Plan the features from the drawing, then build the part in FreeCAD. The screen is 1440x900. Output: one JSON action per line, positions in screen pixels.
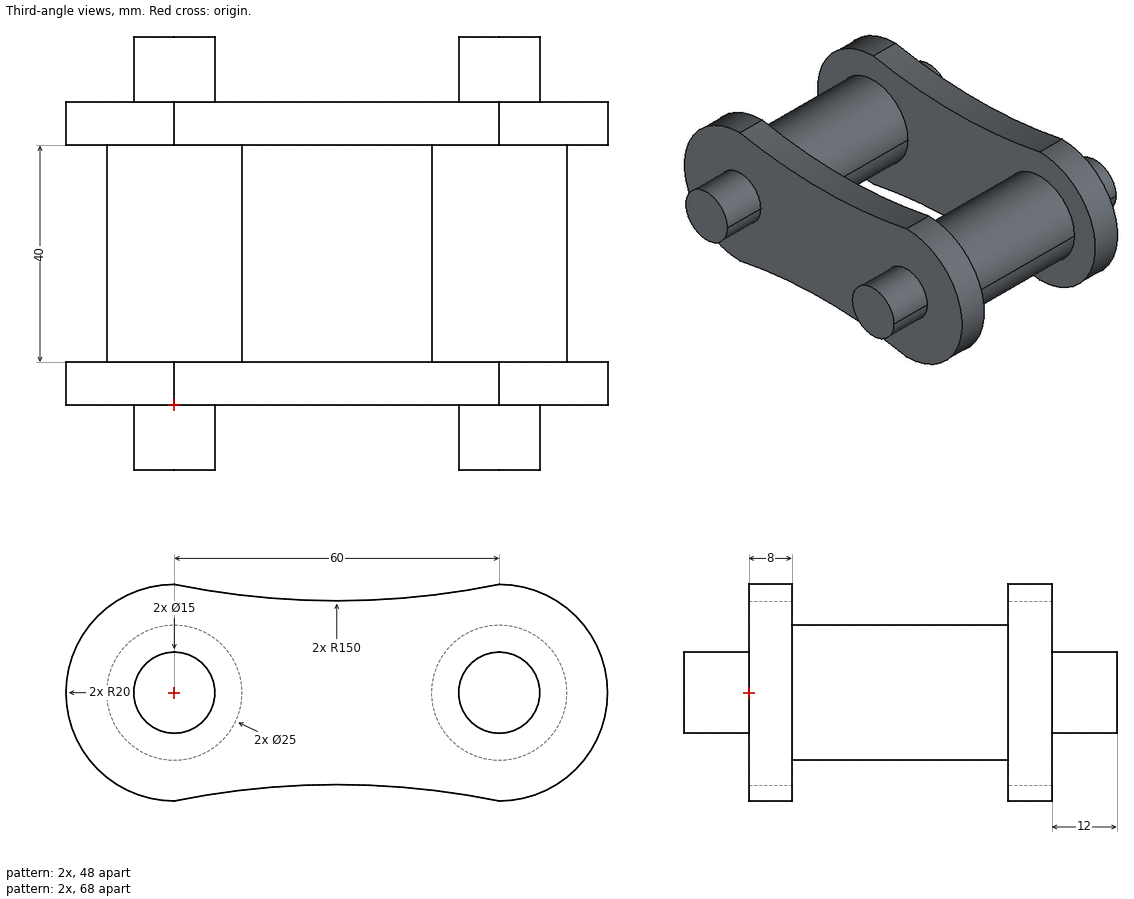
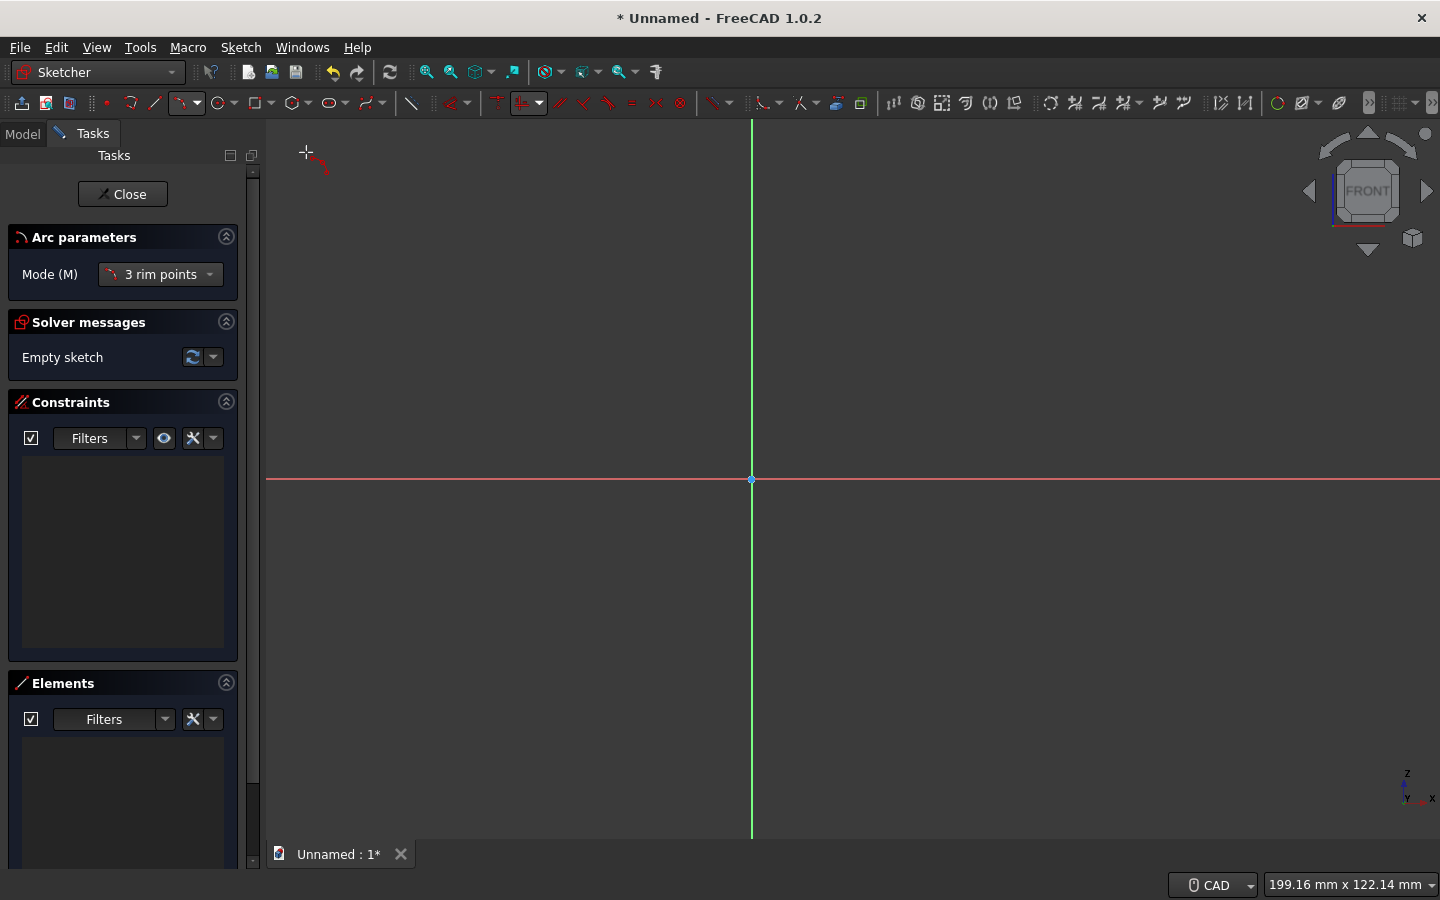
{"action": "left_click", "coordinate": [752, 597]}
{"action": "left_click", "coordinate": [752, 361]}
{"action": "left_click", "coordinate": [640, 443]}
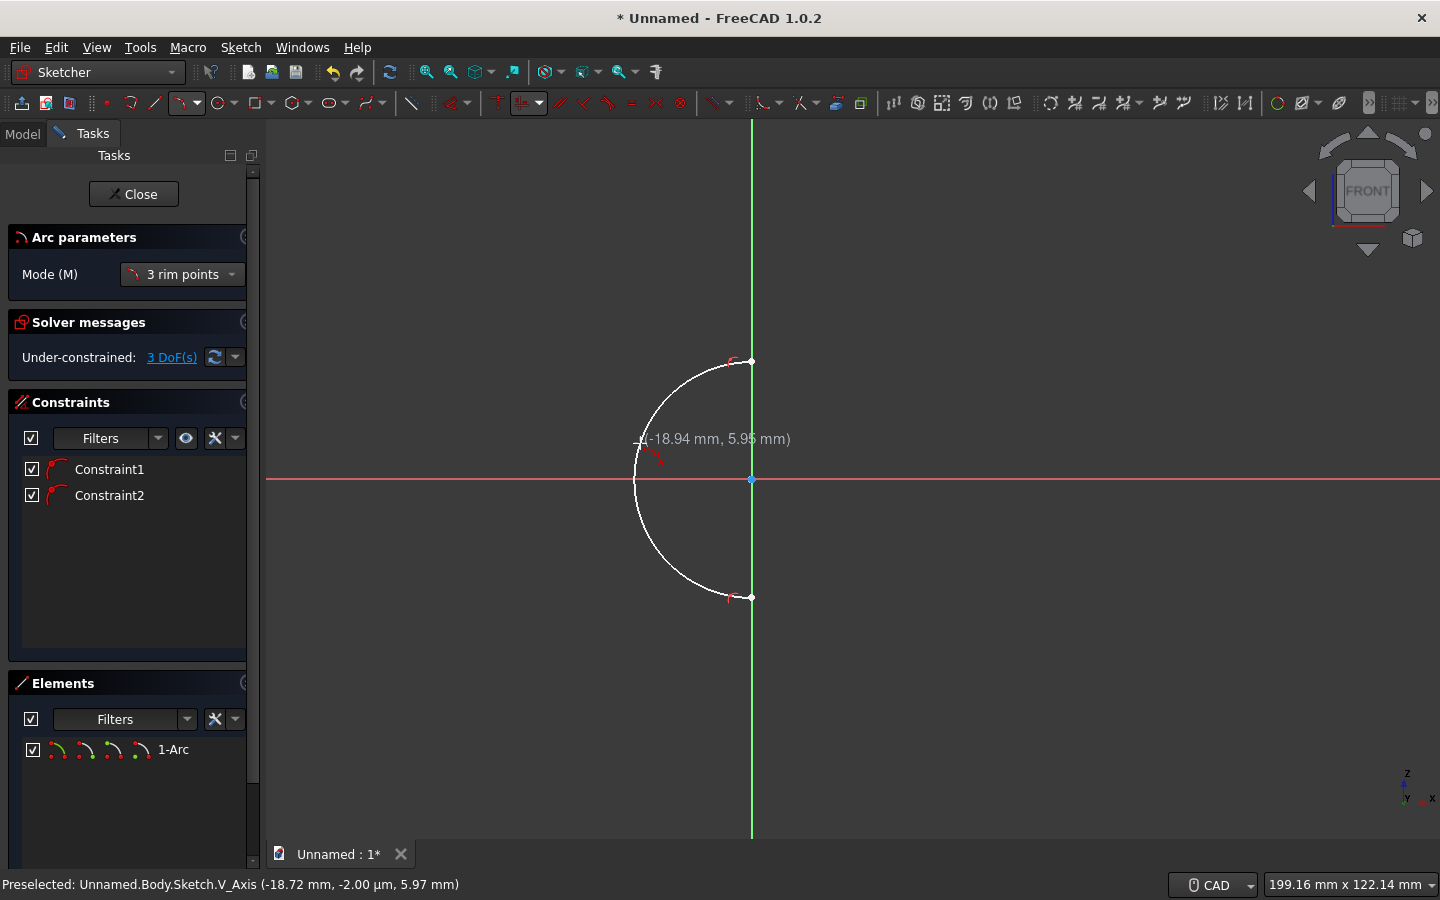
{"action": "left_click", "coordinate": [752, 362]}
{"action": "left_click", "coordinate": [1105, 361]}
{"action": "left_click", "coordinate": [929, 379]}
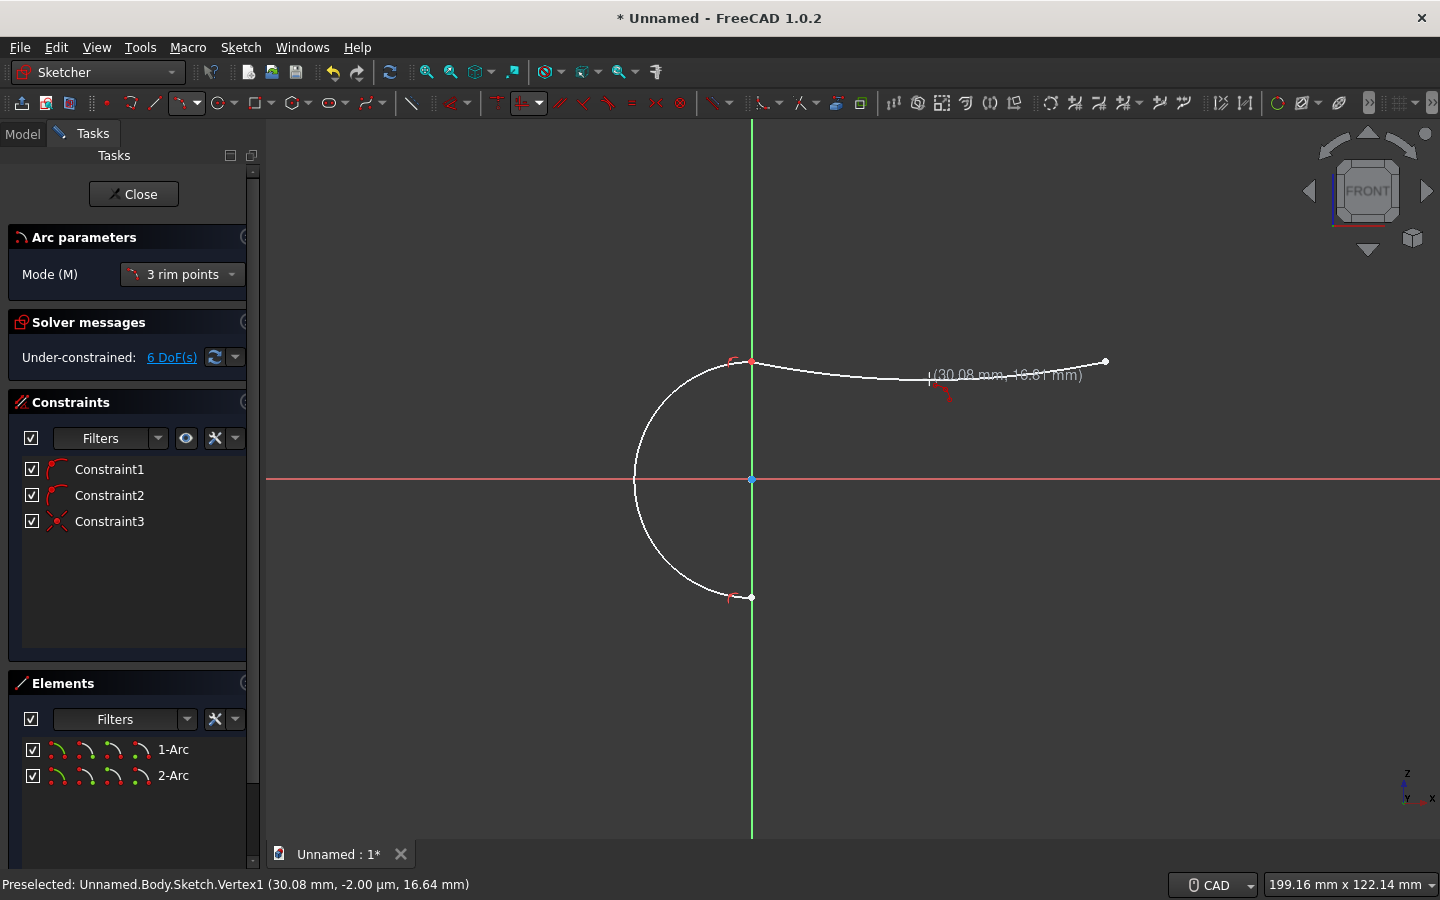
{"action": "left_click", "coordinate": [1105, 362]}
{"action": "left_click", "coordinate": [1105, 597]}
{"action": "left_click", "coordinate": [1217, 516]}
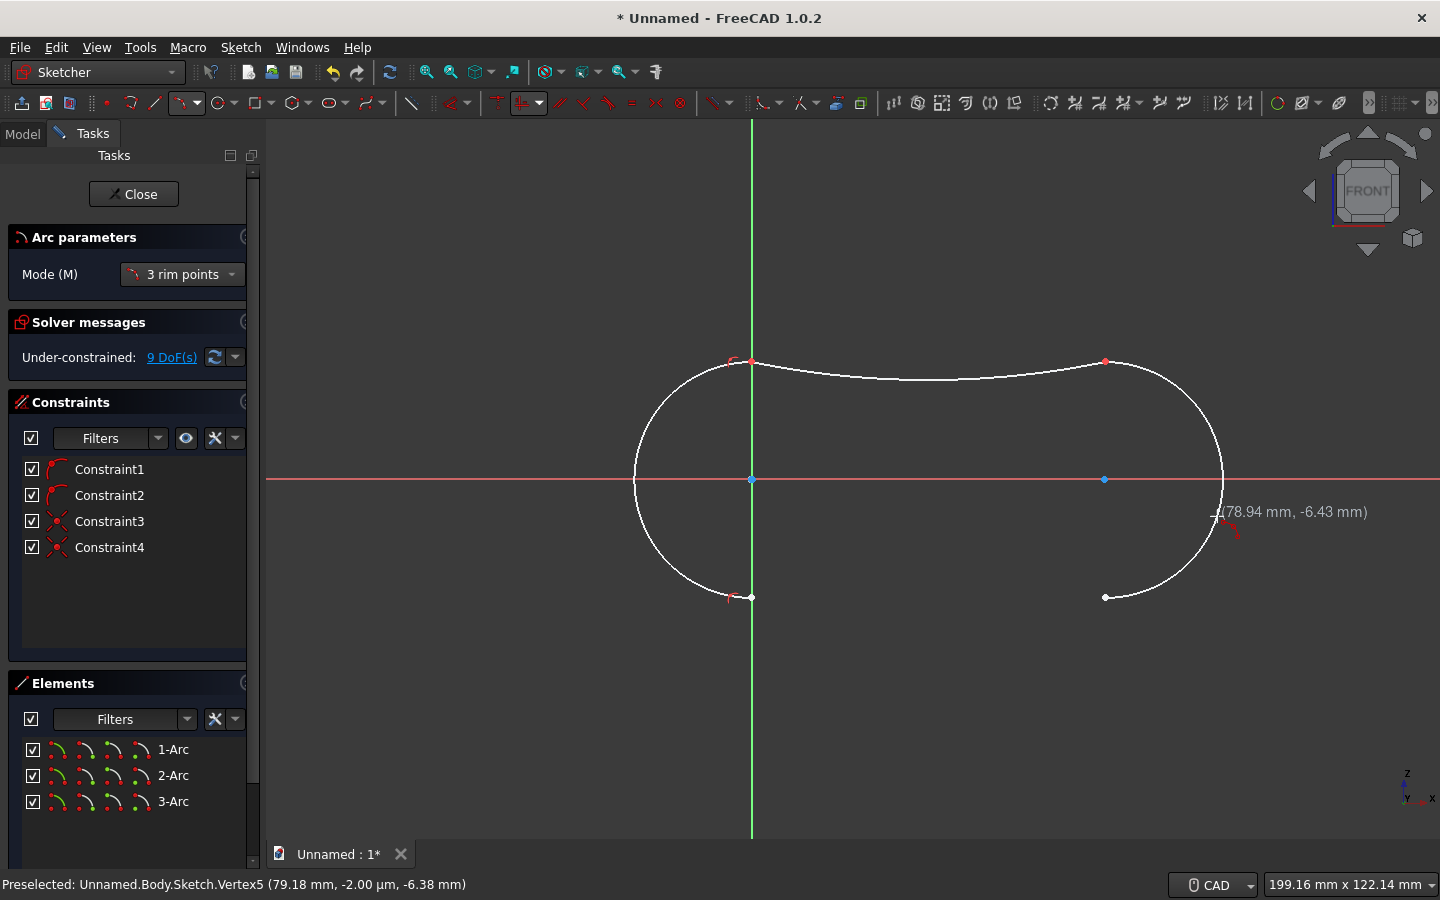
{"action": "left_click", "coordinate": [1105, 598]}
{"action": "left_click", "coordinate": [752, 598]}
{"action": "left_click", "coordinate": [929, 579]}
{"action": "key", "text": "Escape"}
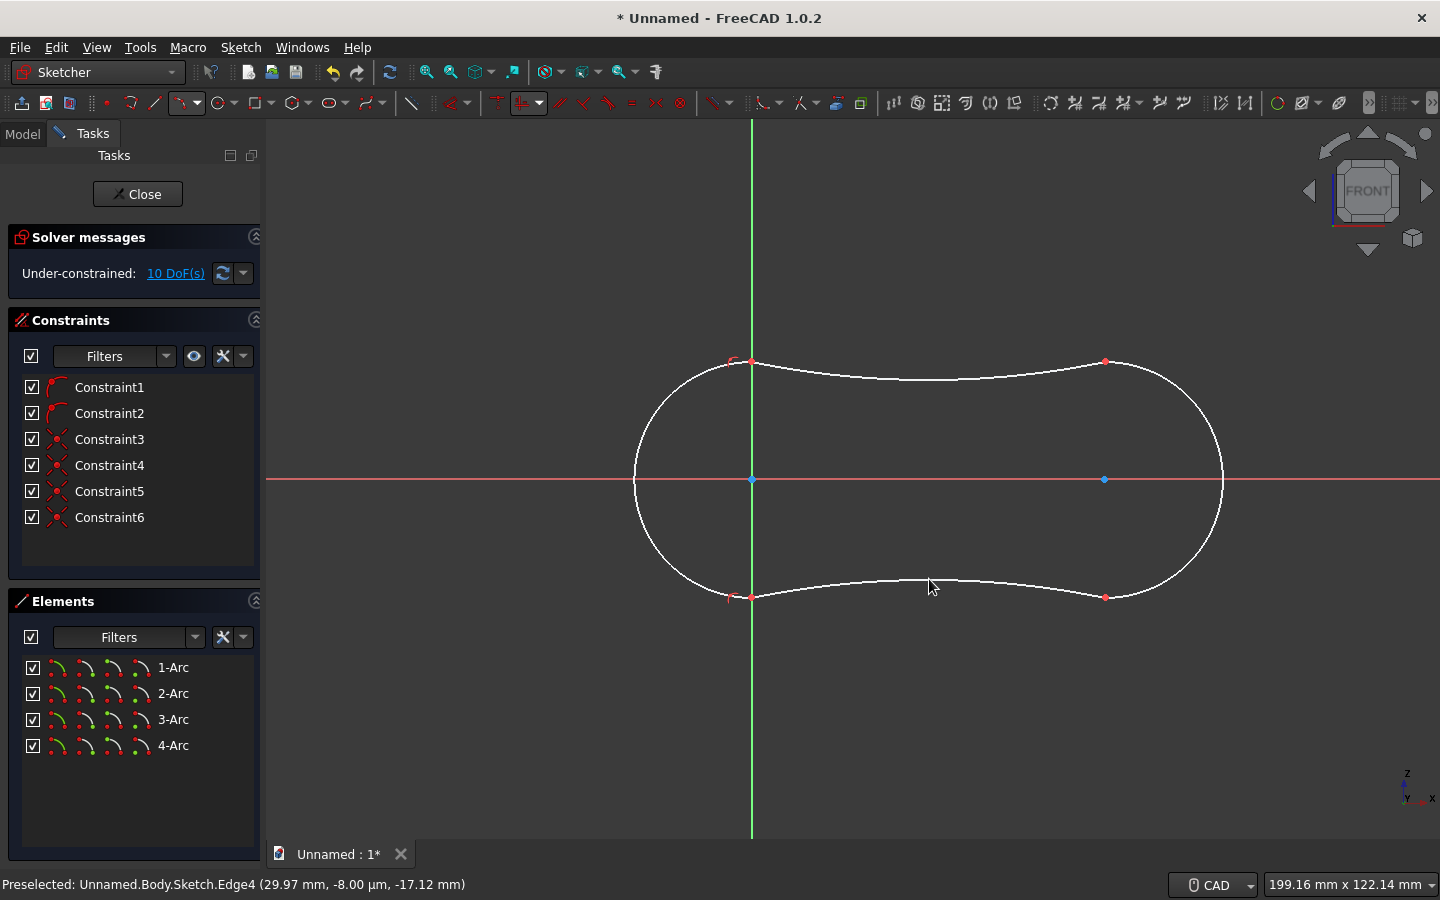
{"action": "left_click_drag", "start_coordinate": [742, 469], "coordinate": [762, 490]}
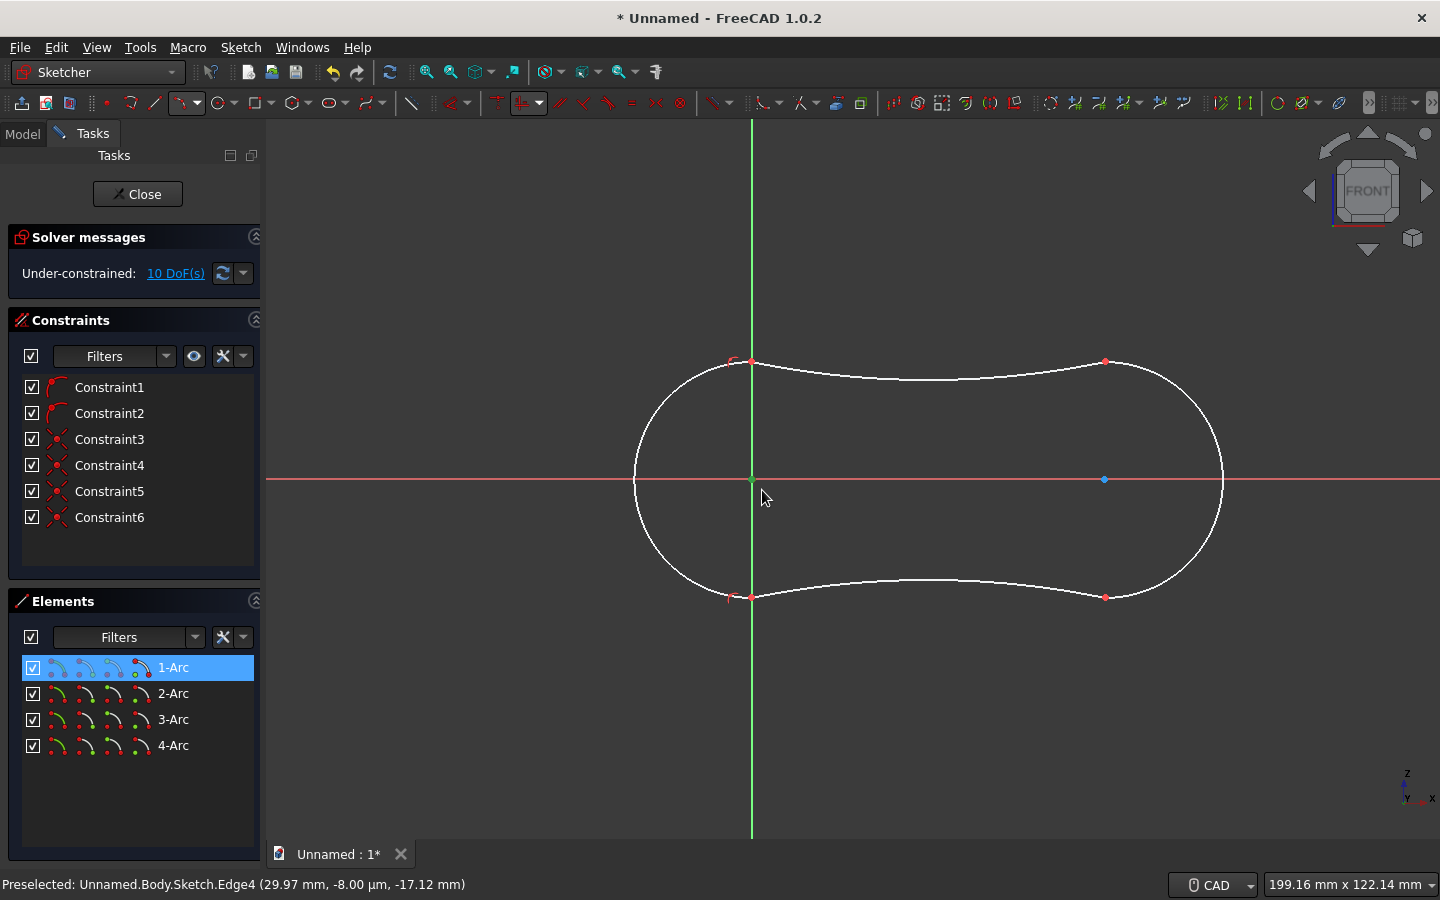
{"action": "left_click", "coordinate": [498, 104]}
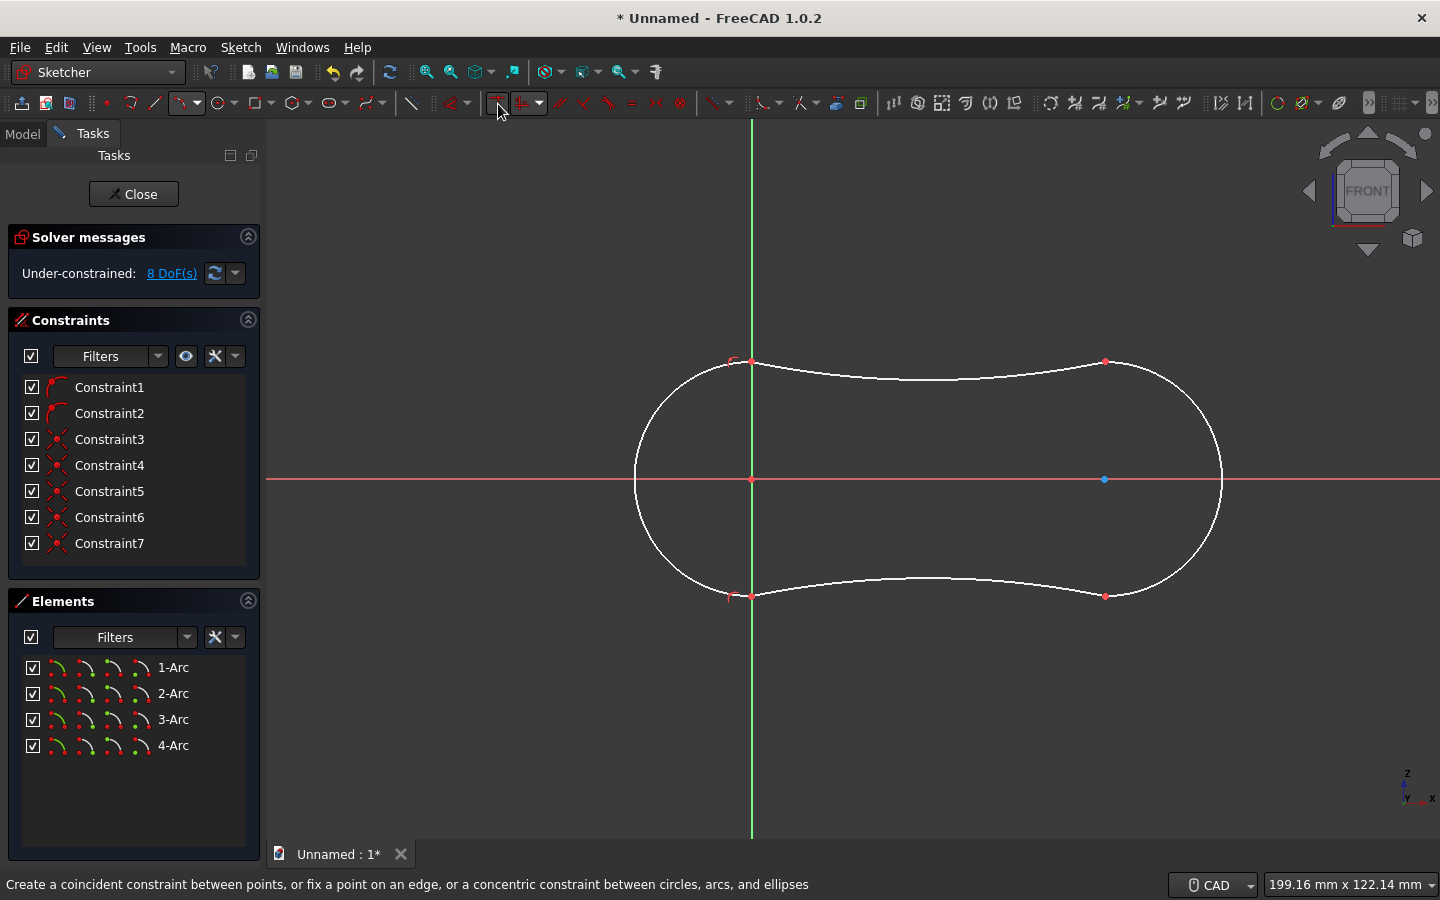
{"action": "left_click", "coordinate": [657, 410]}